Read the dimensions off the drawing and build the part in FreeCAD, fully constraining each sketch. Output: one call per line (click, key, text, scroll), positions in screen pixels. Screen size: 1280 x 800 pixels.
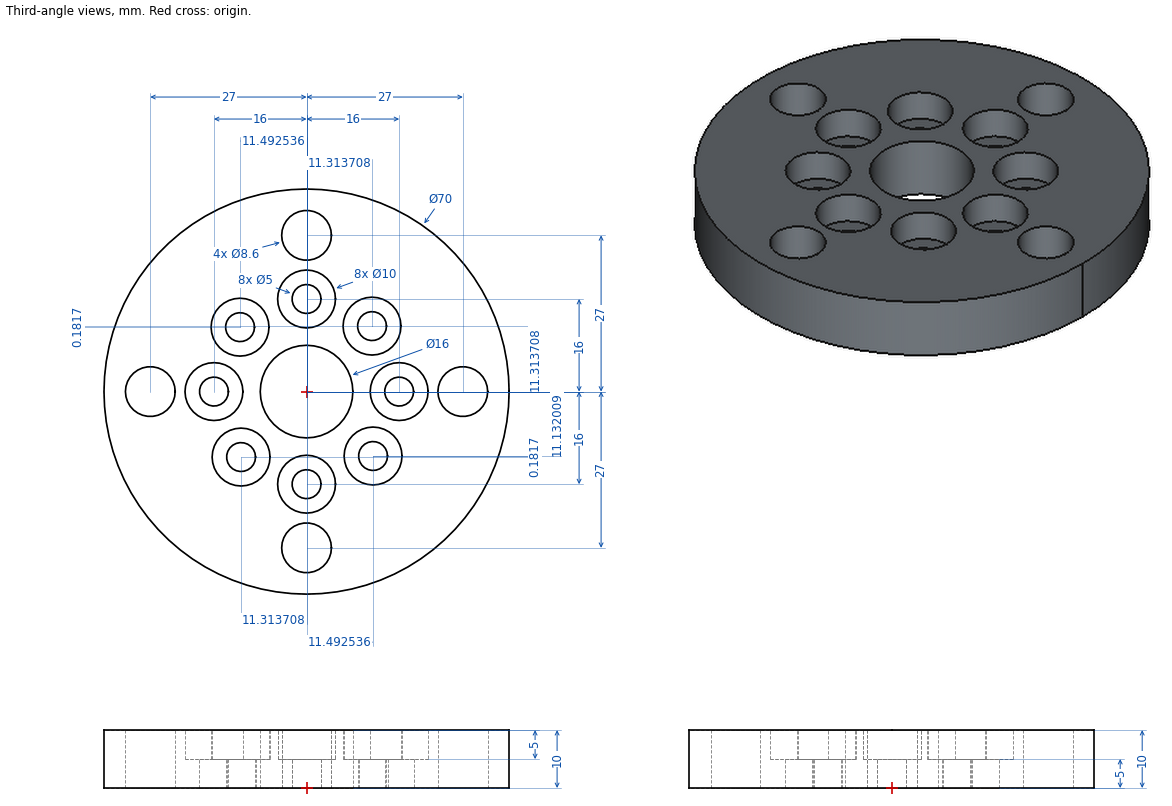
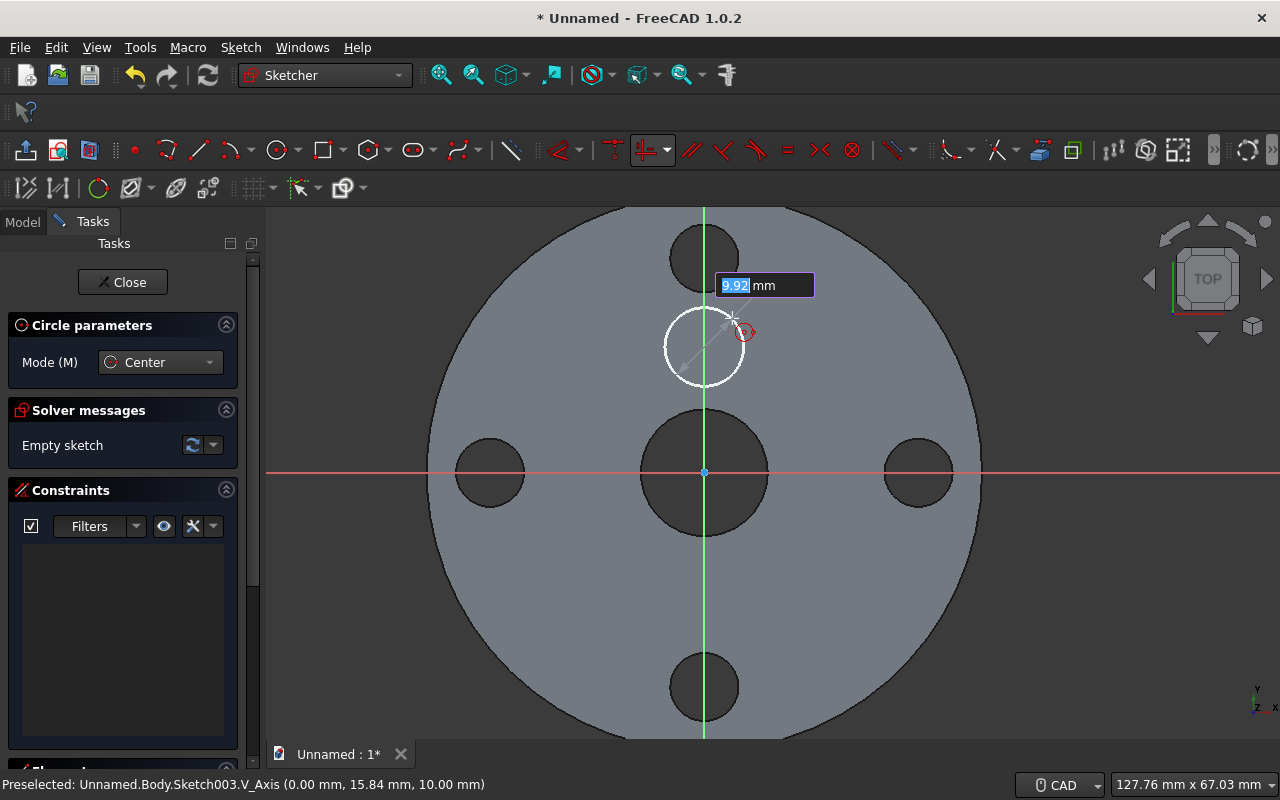
text(10)
key(Return)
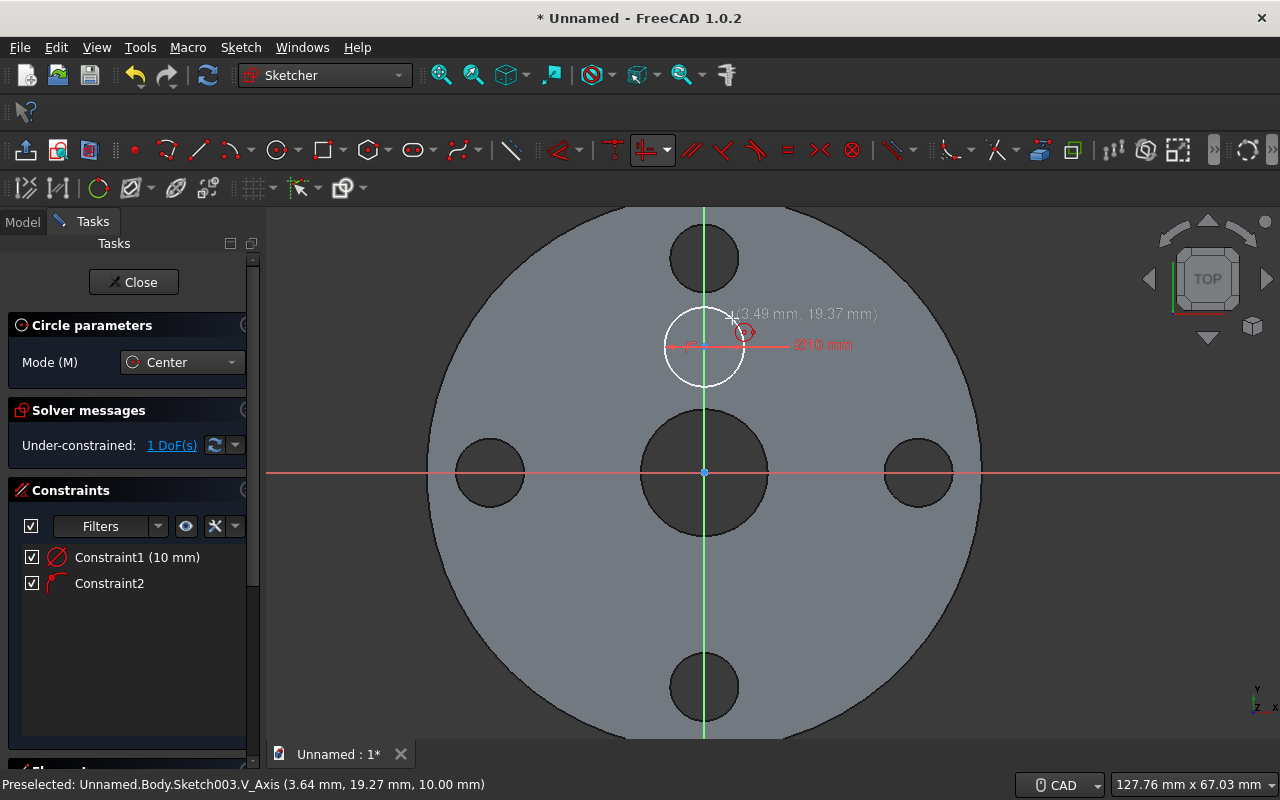
click(831, 473)
move(859, 445)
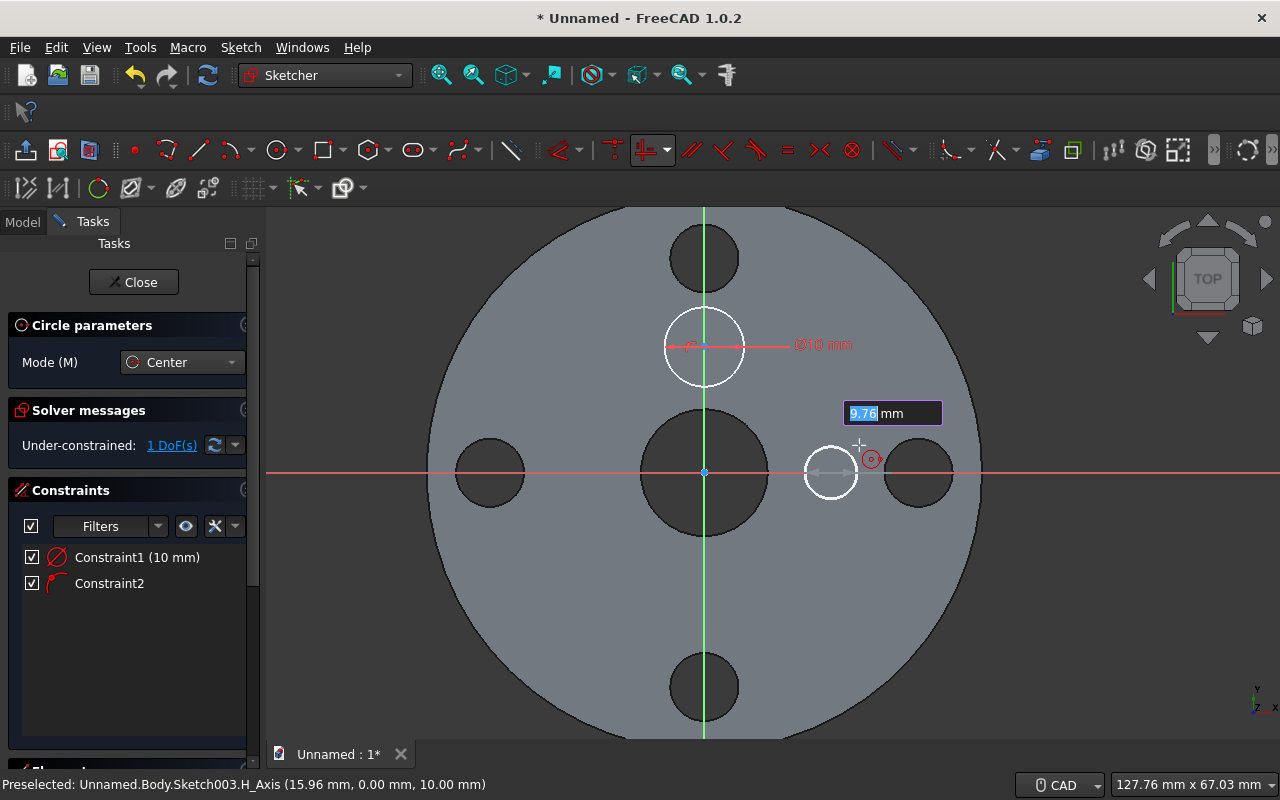
text(10)
key(Return)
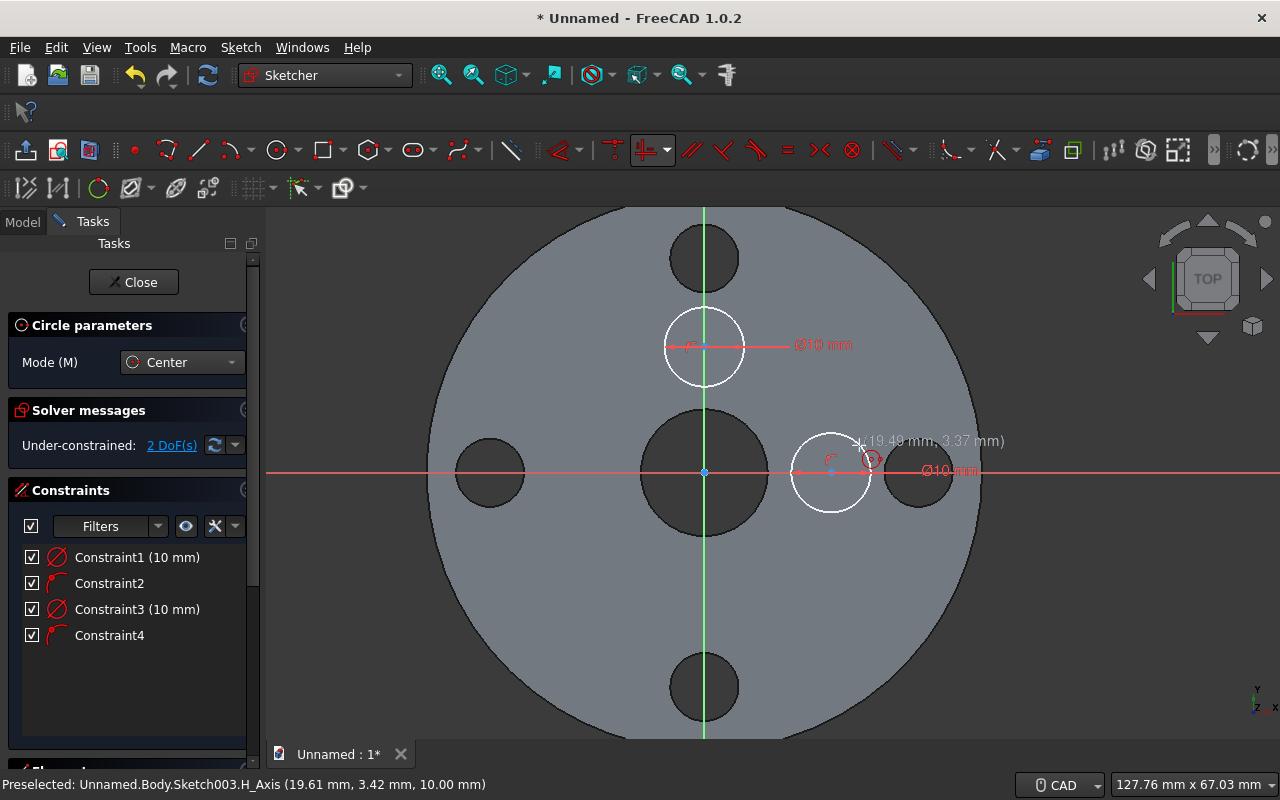
click(704, 600)
move(732, 572)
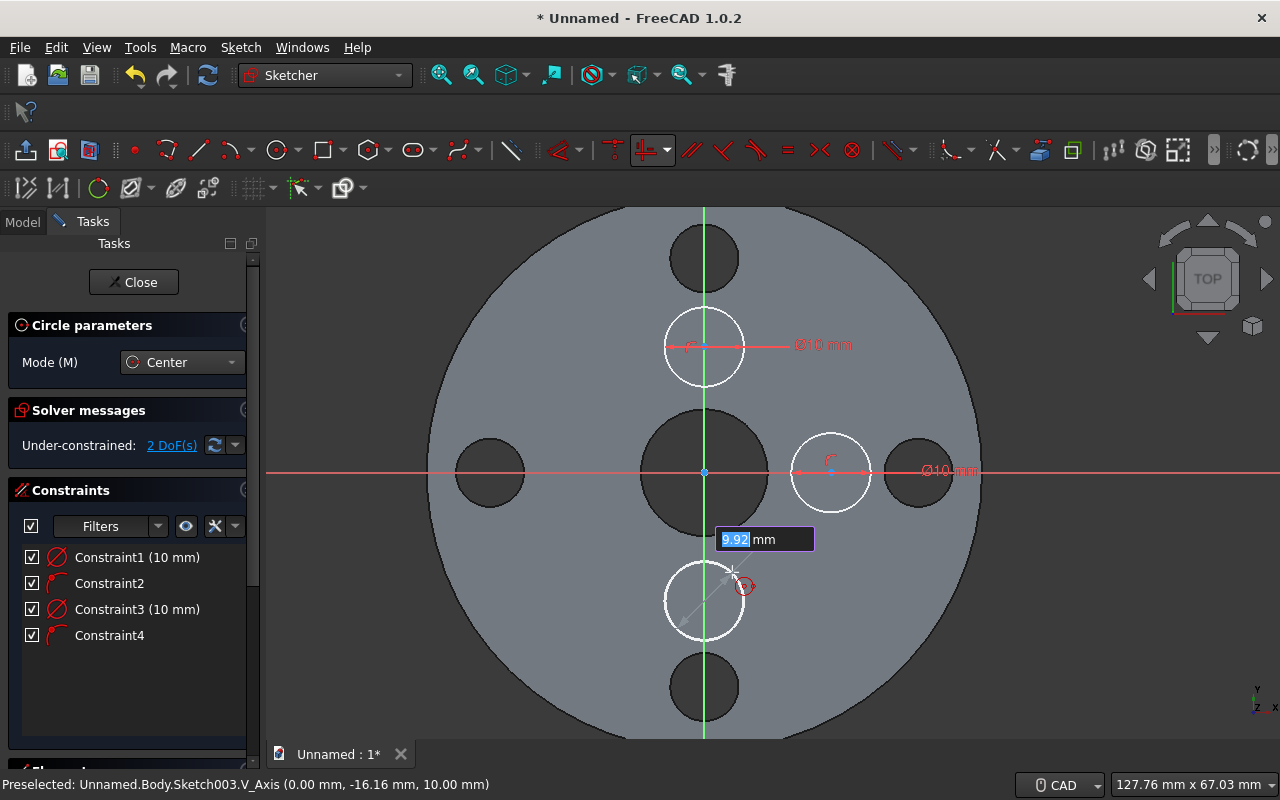
text(10)
key(Return)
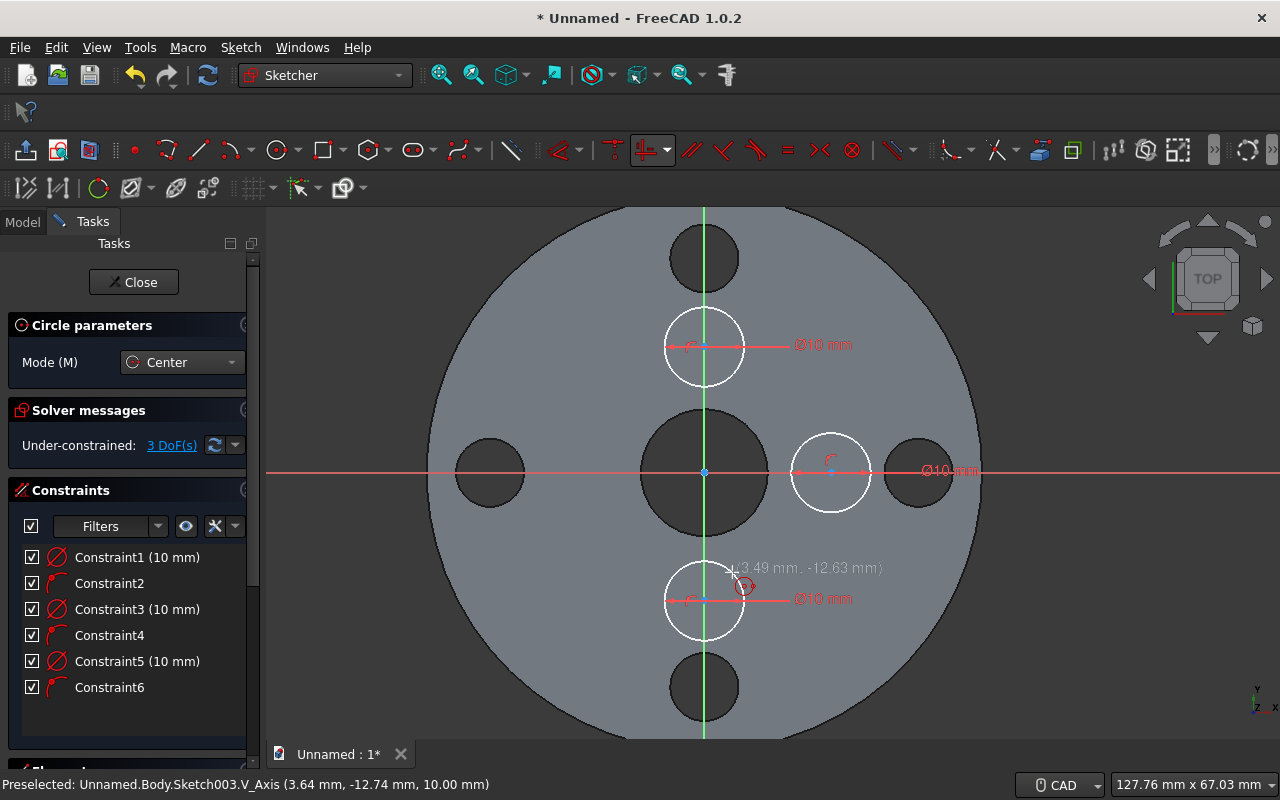
click(577, 473)
move(605, 445)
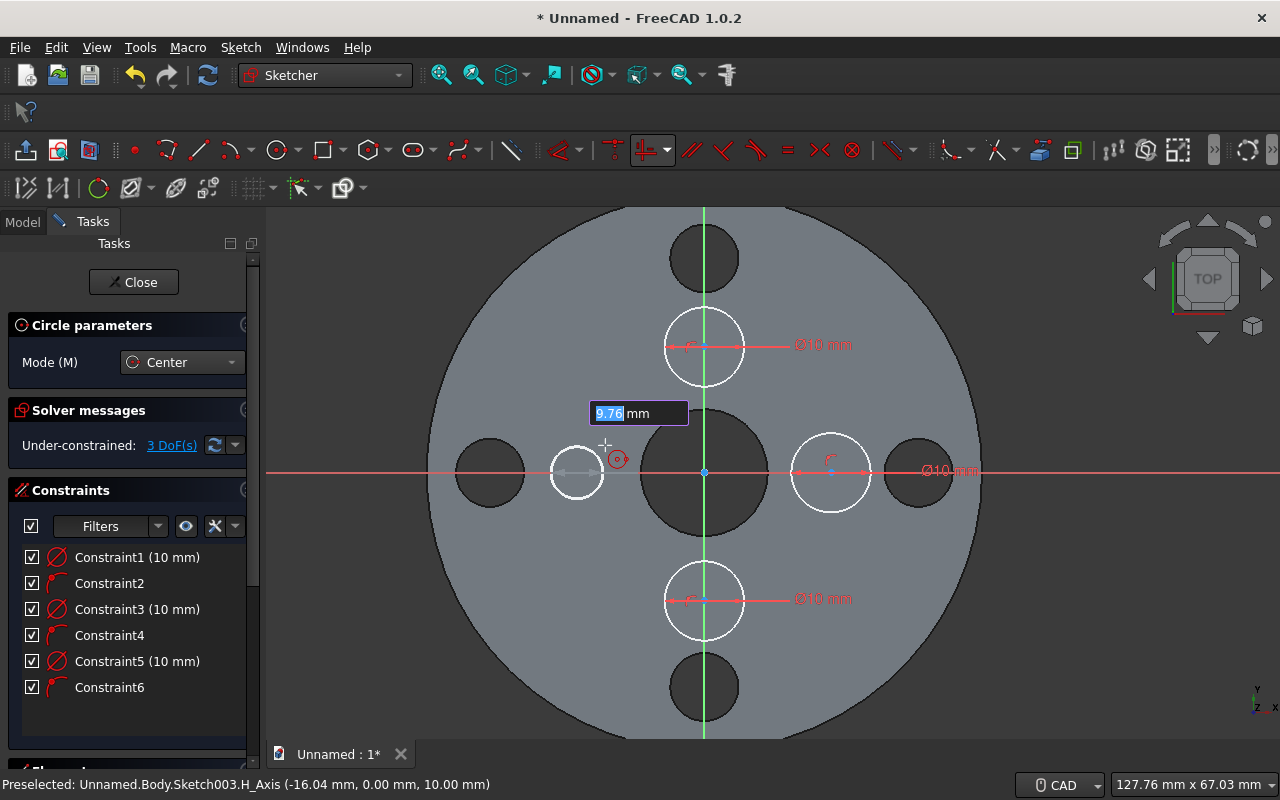
text(10)
key(Return)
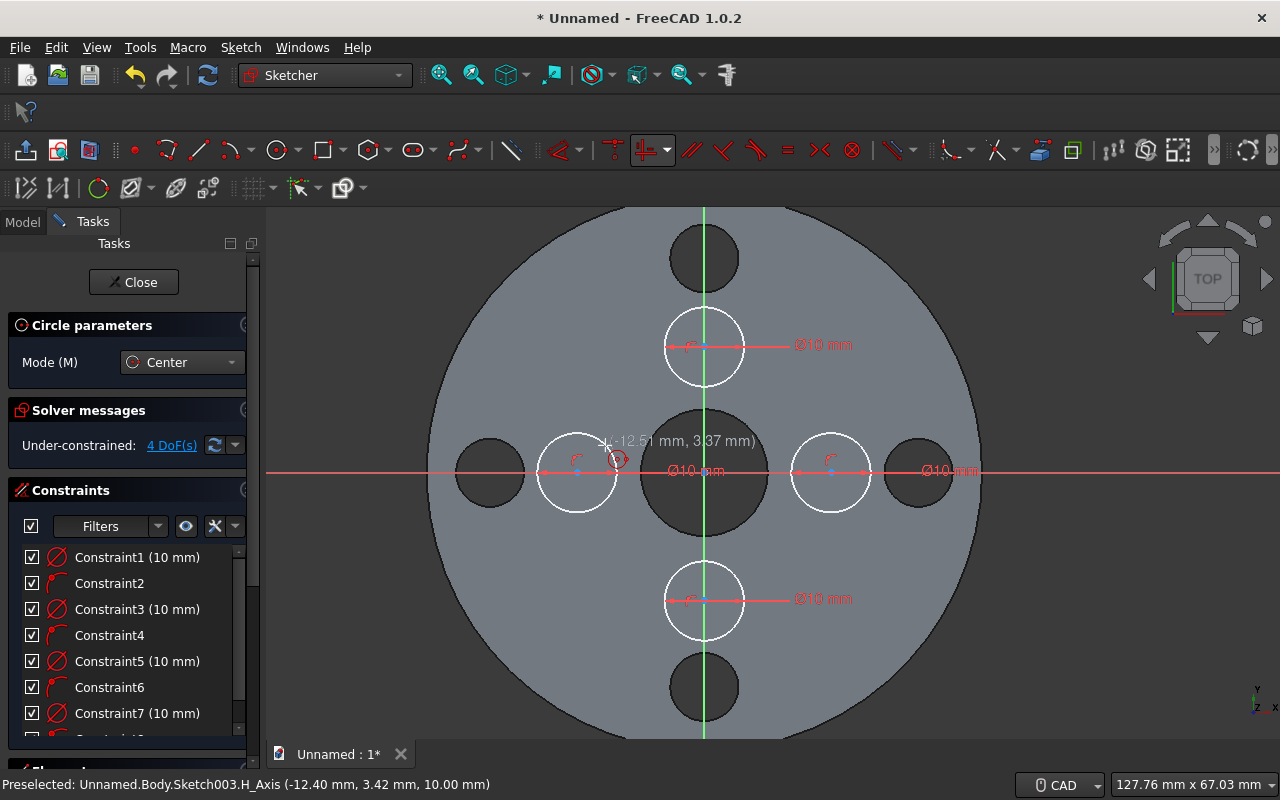
click(796, 561)
move(824, 533)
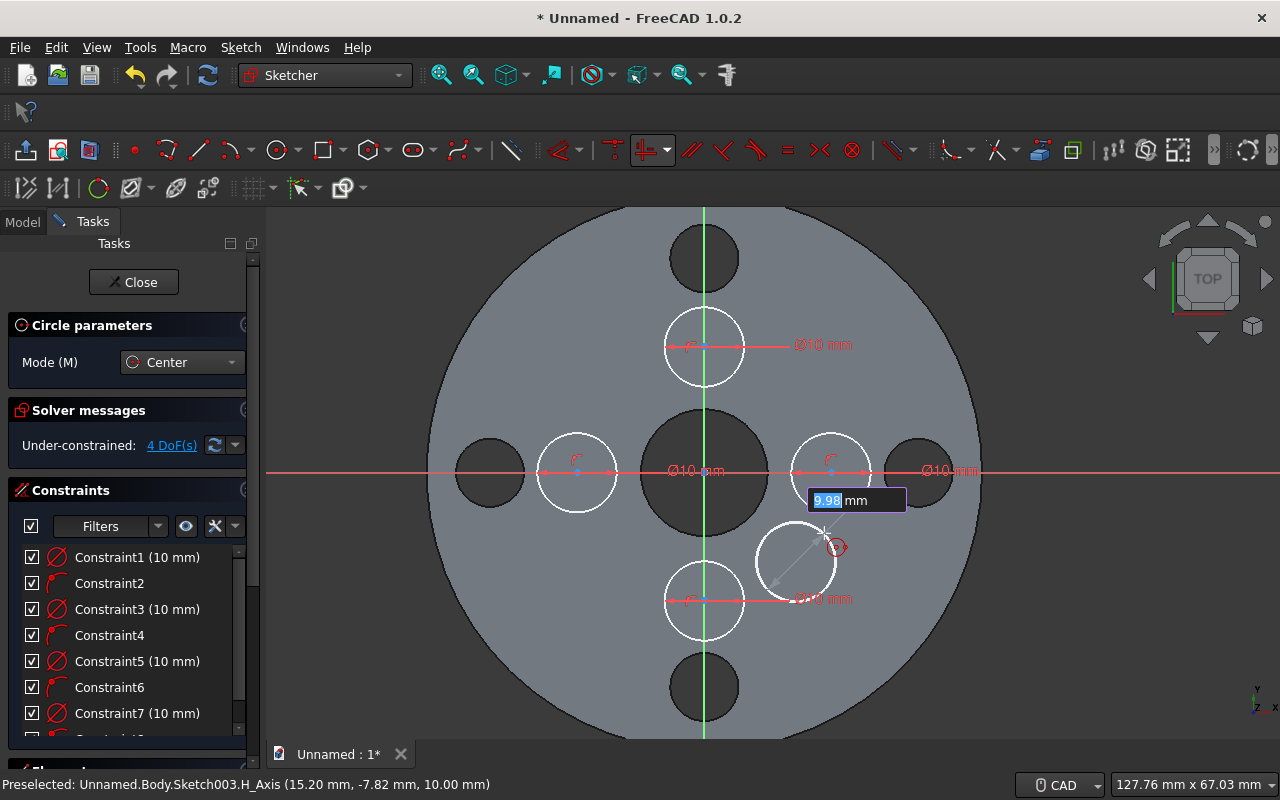
text(10)
key(Return)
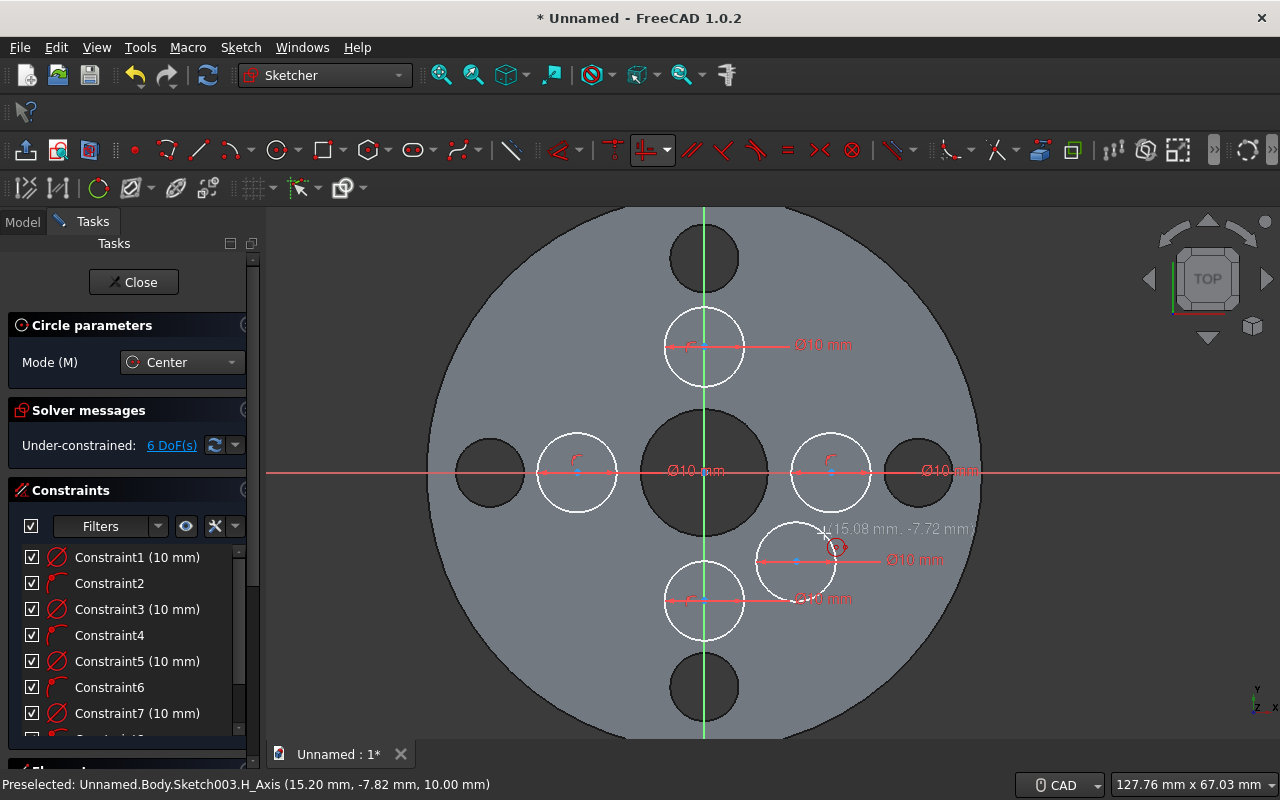
click(794, 383)
move(822, 355)